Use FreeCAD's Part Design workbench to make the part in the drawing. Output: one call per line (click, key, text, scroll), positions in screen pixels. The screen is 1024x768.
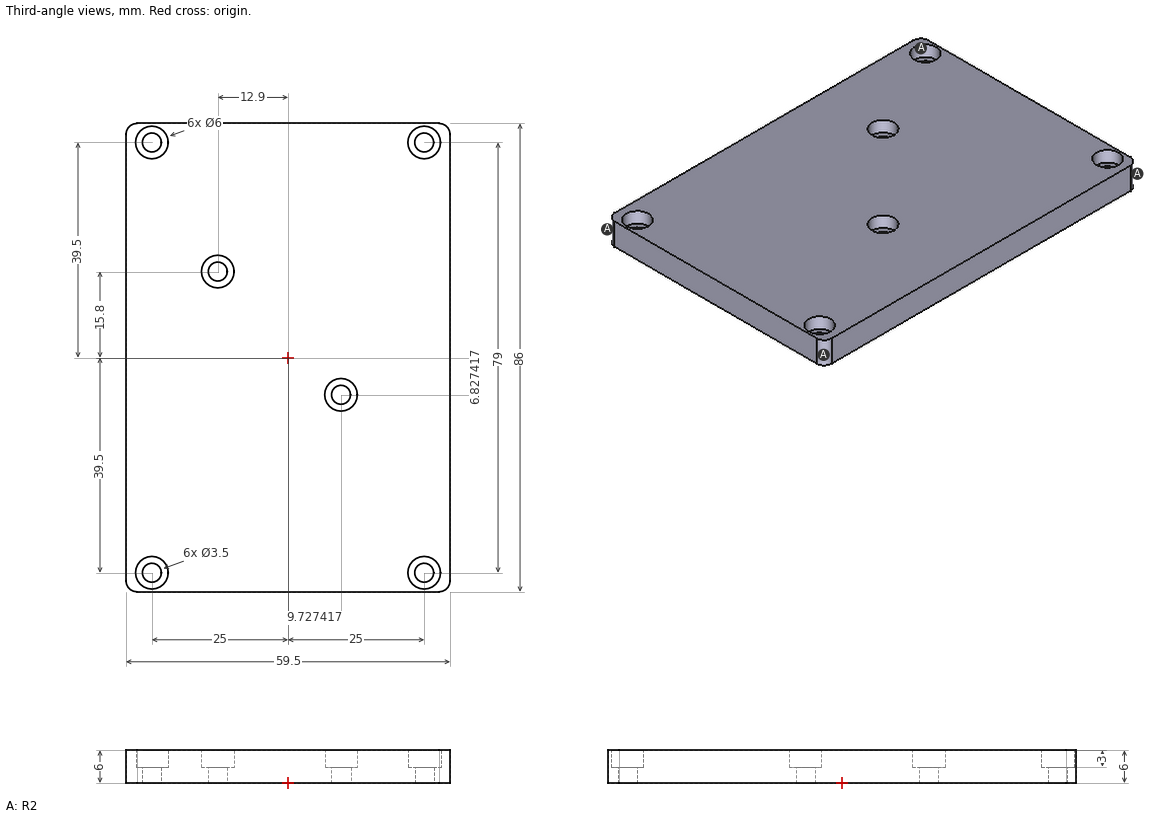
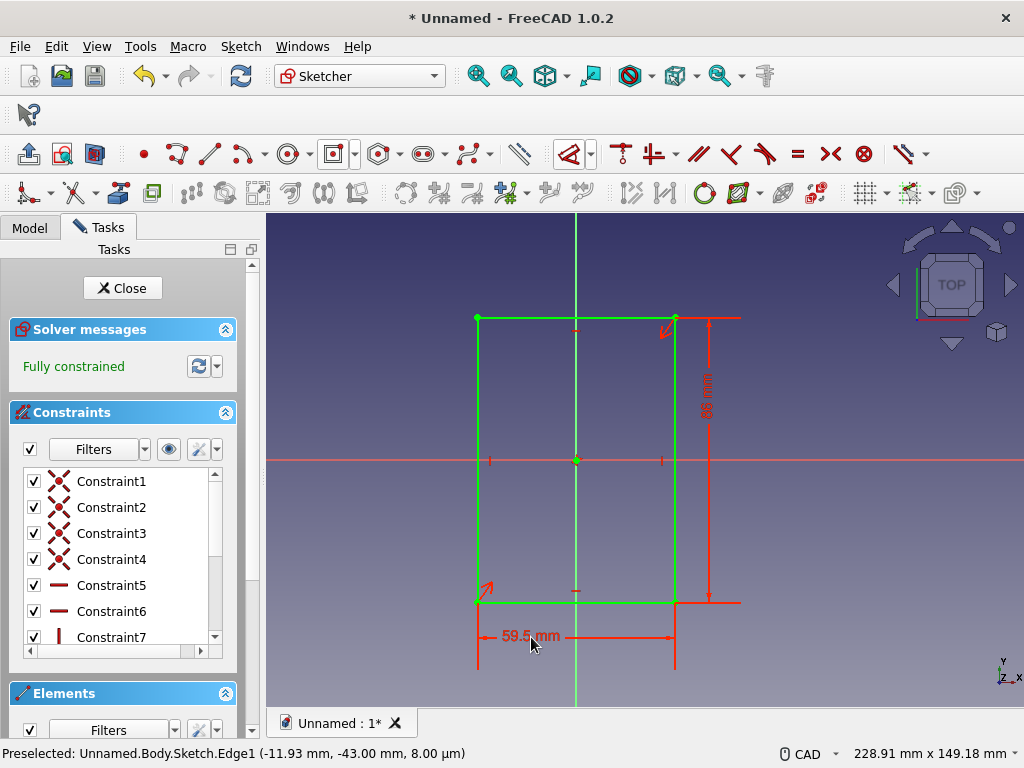
click(123, 288)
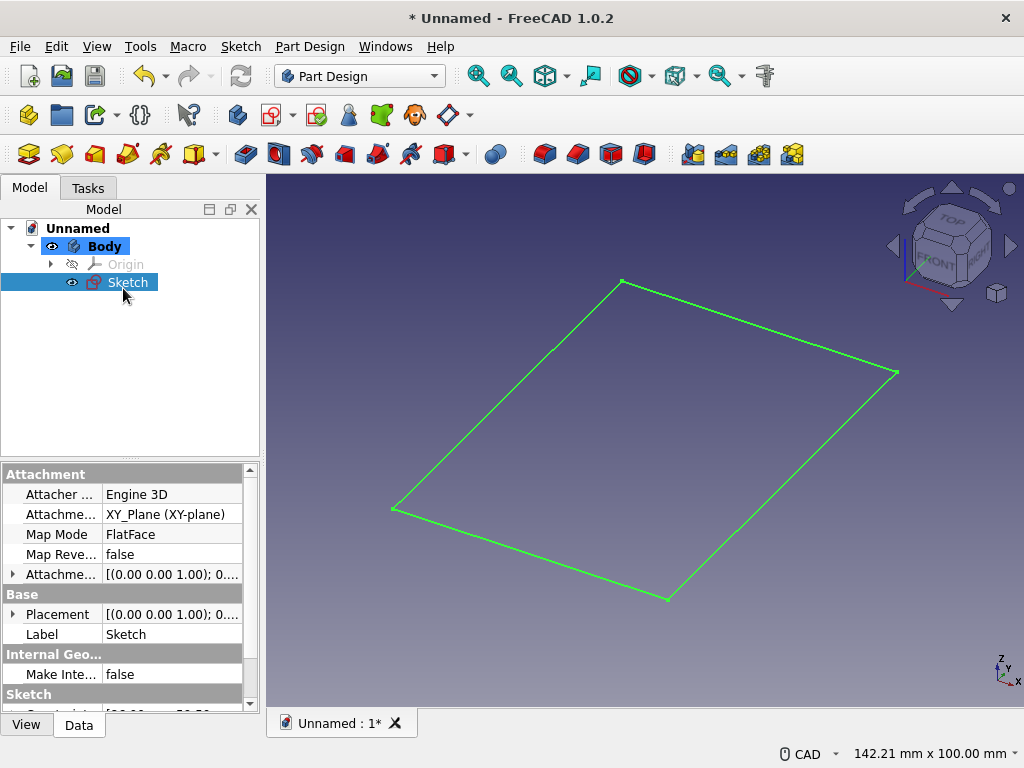
click(29, 154)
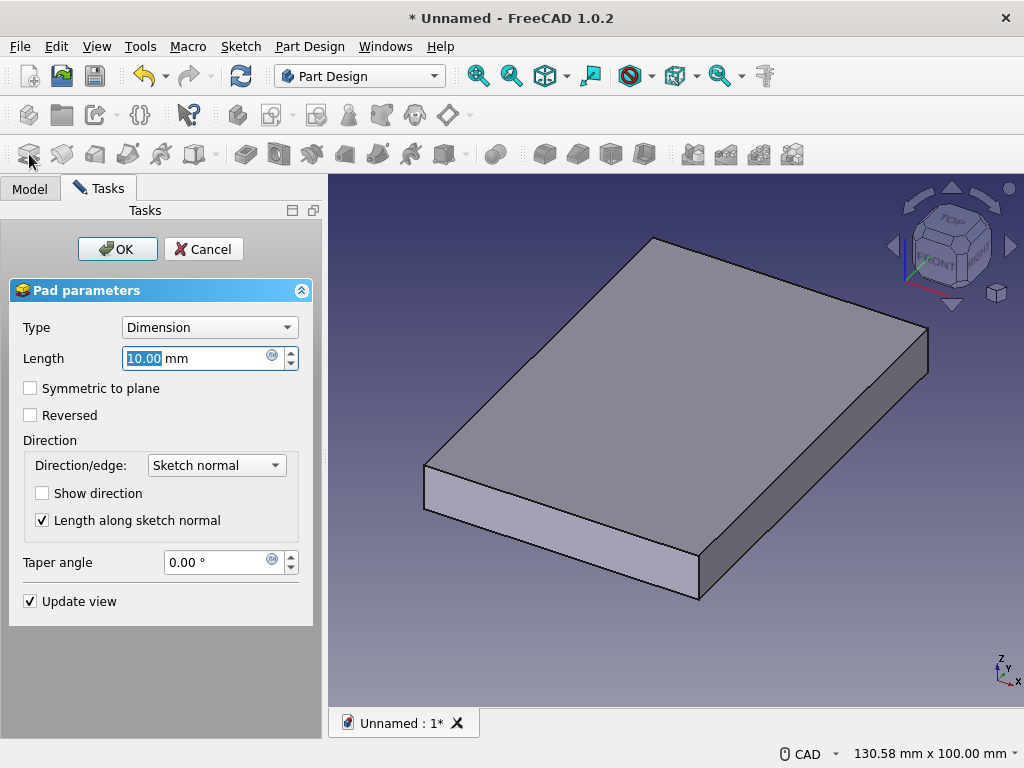
text(6)
key(Tab)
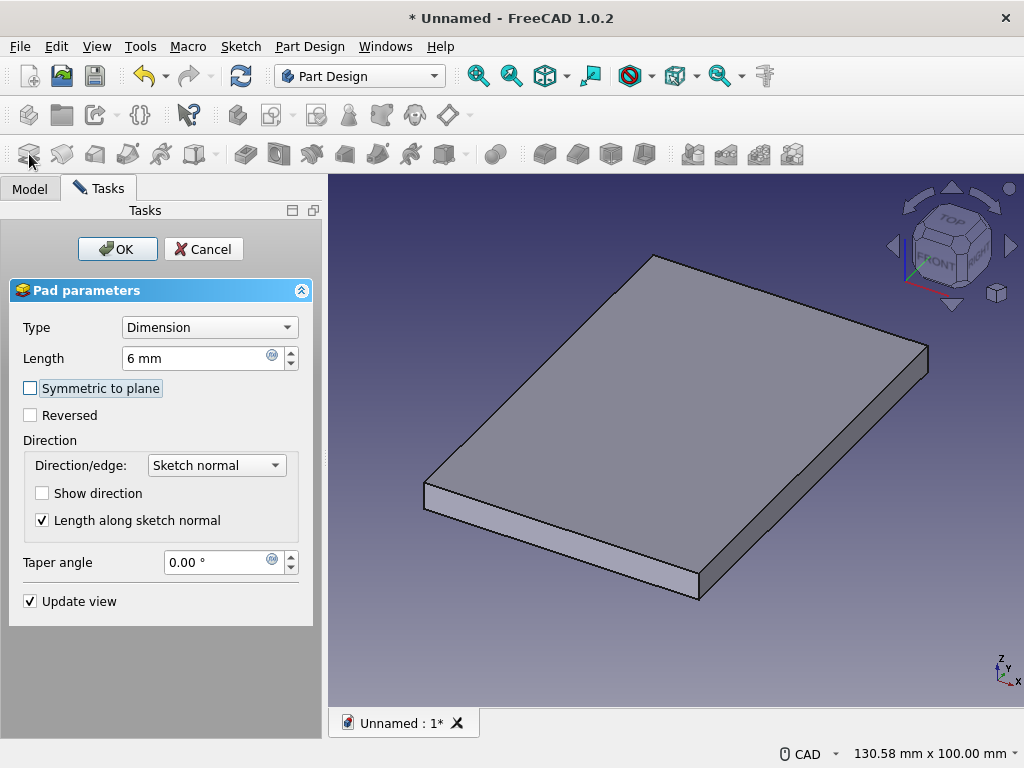
click(118, 249)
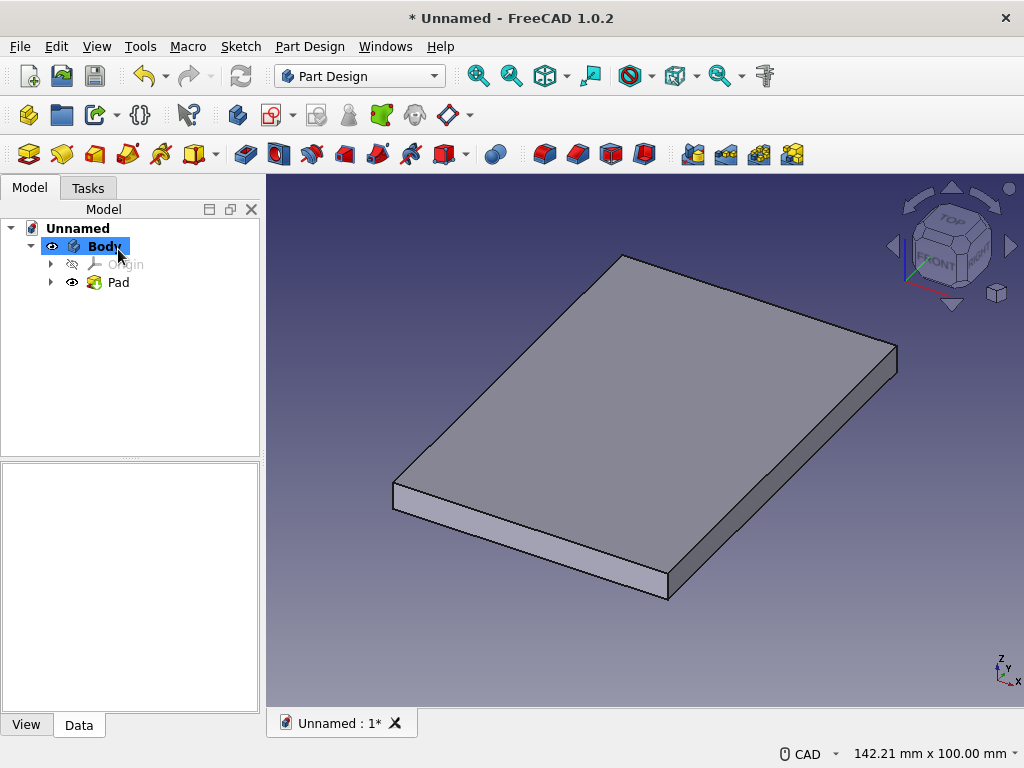
click(678, 381)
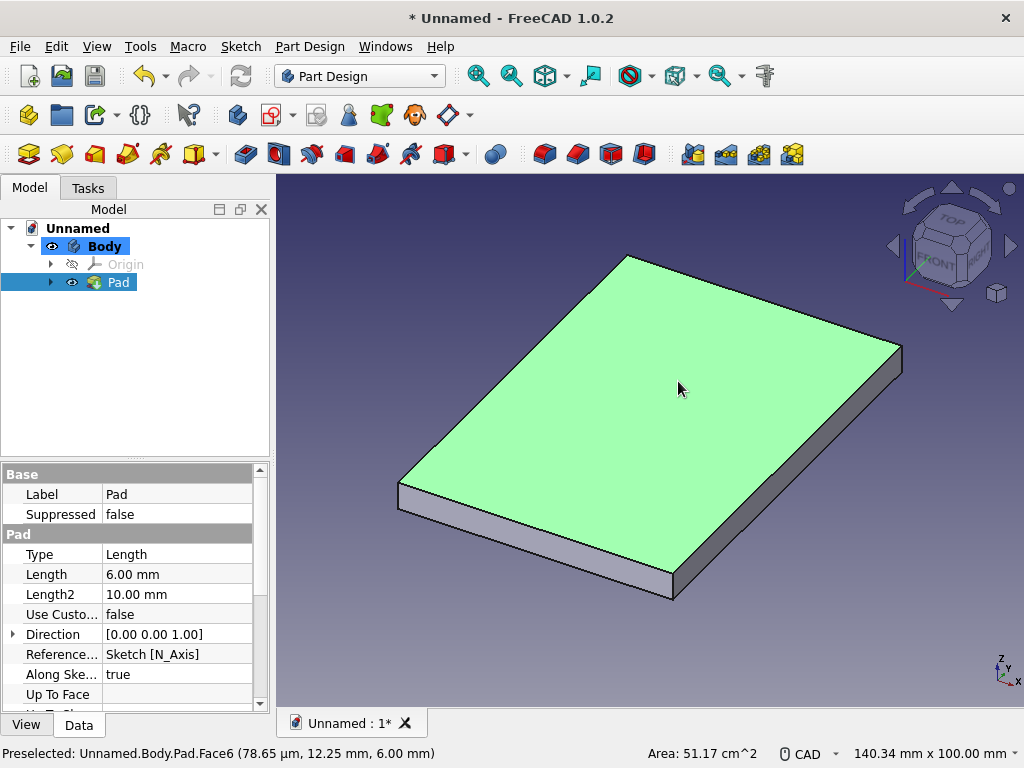
click(270, 116)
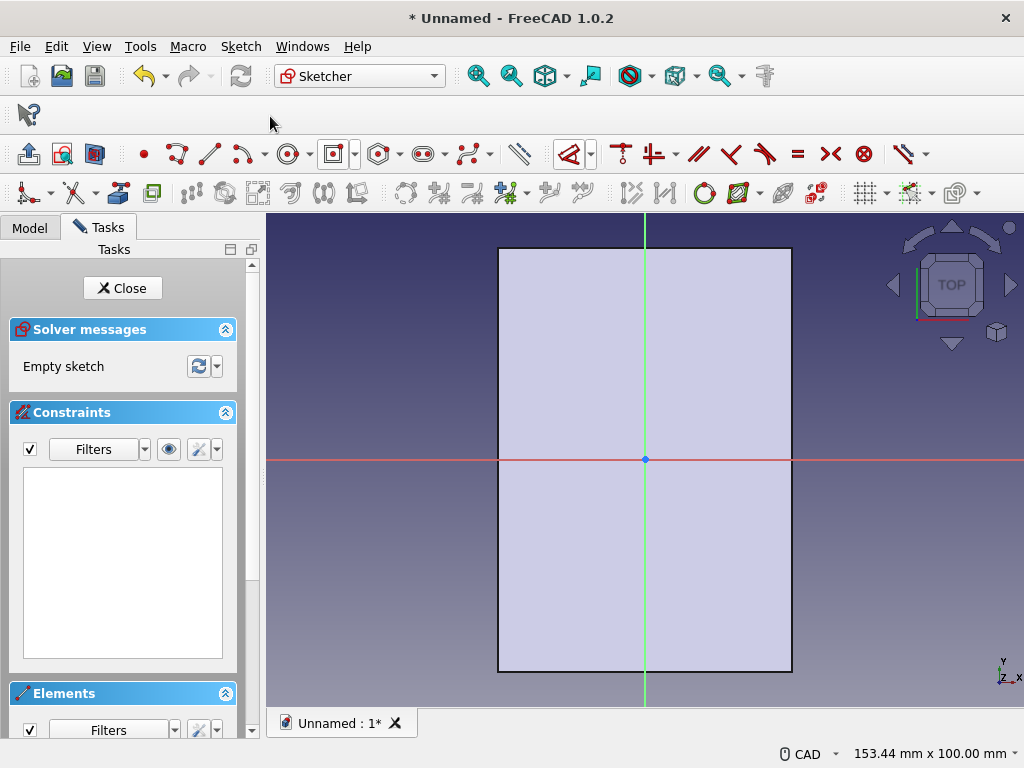
scroll(294, 460, down, 1)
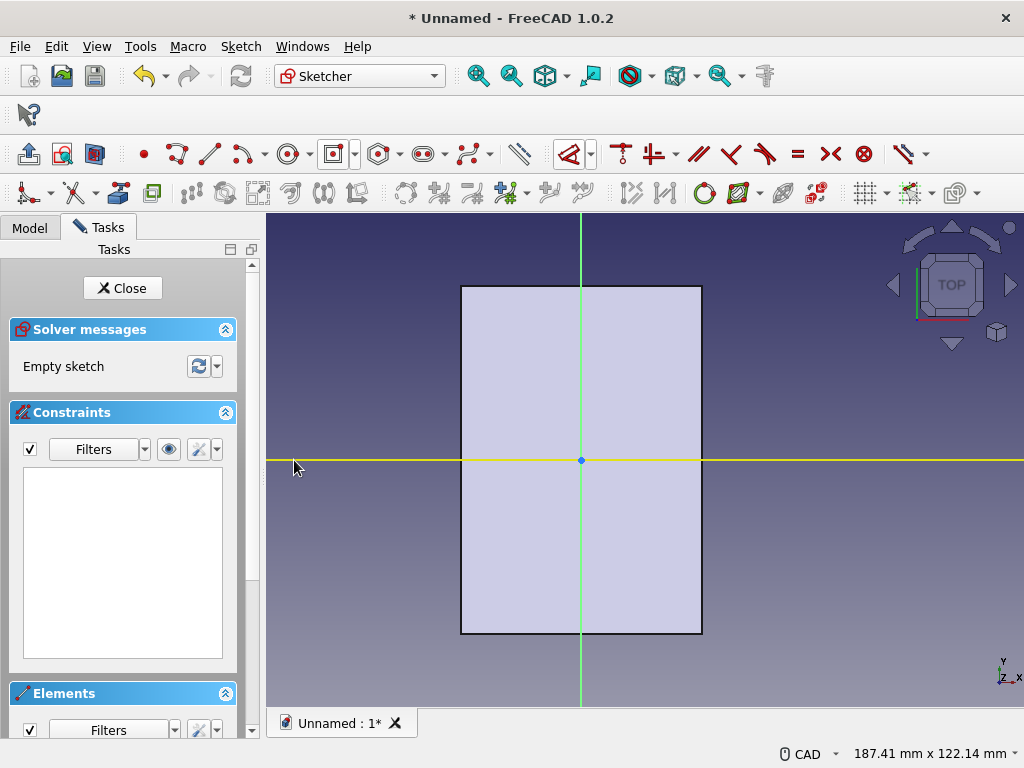
key(g)
key(c)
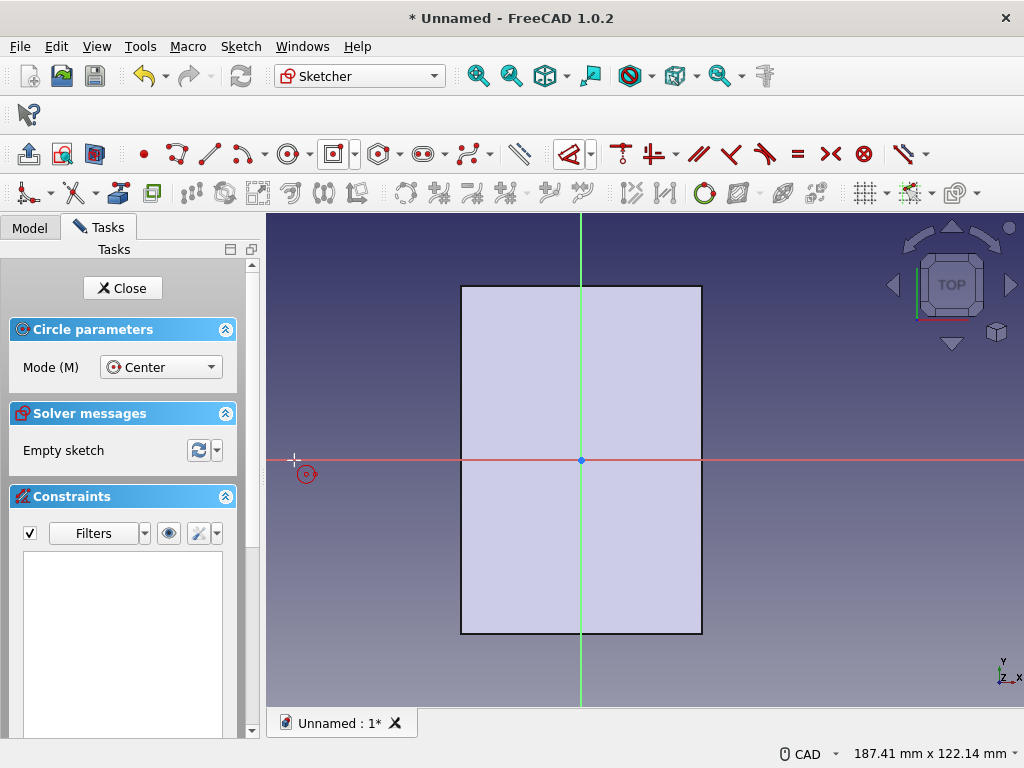
scroll(480, 620, up, 6)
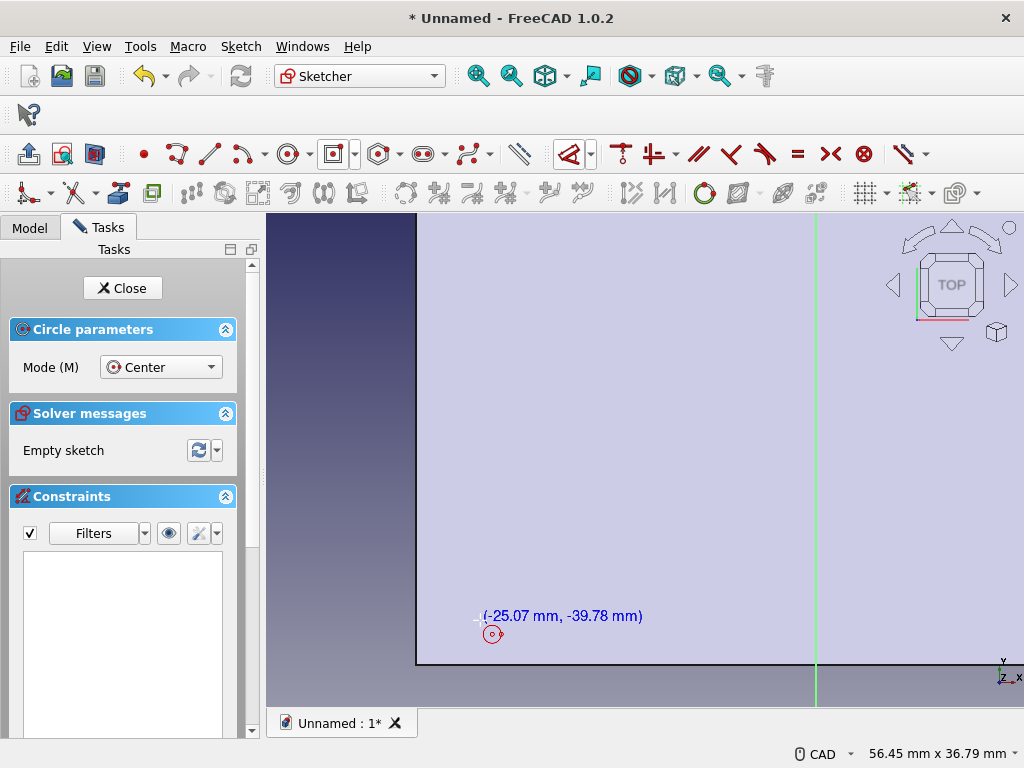
click(480, 618)
click(497, 601)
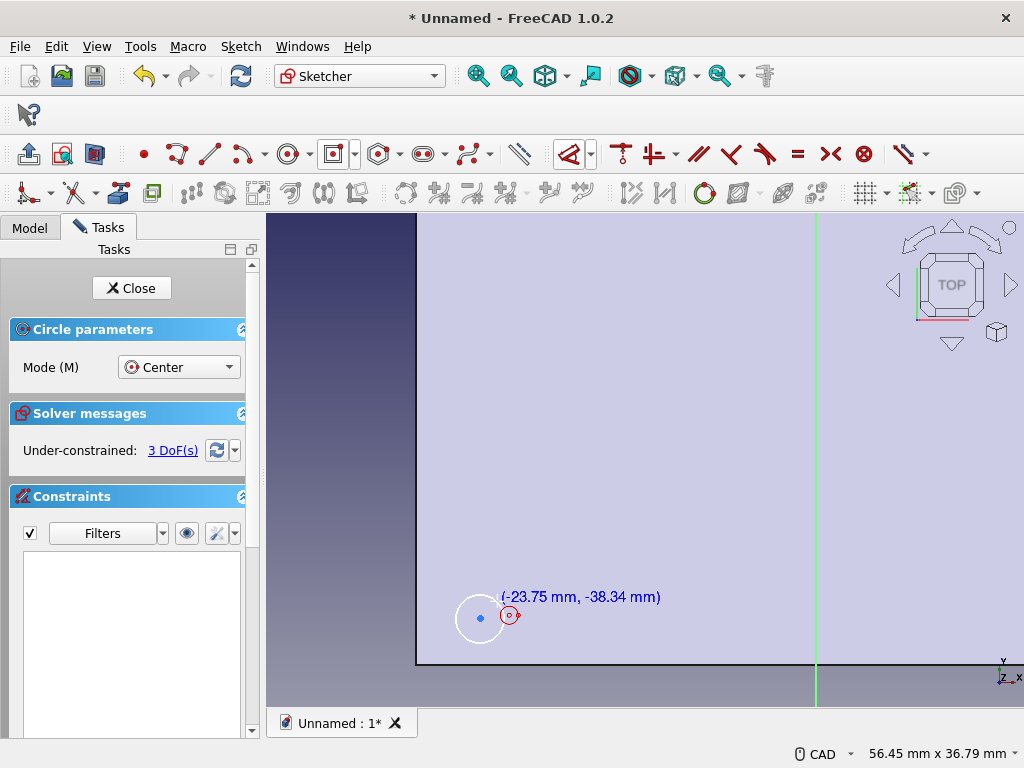
scroll(473, 621, down, 6)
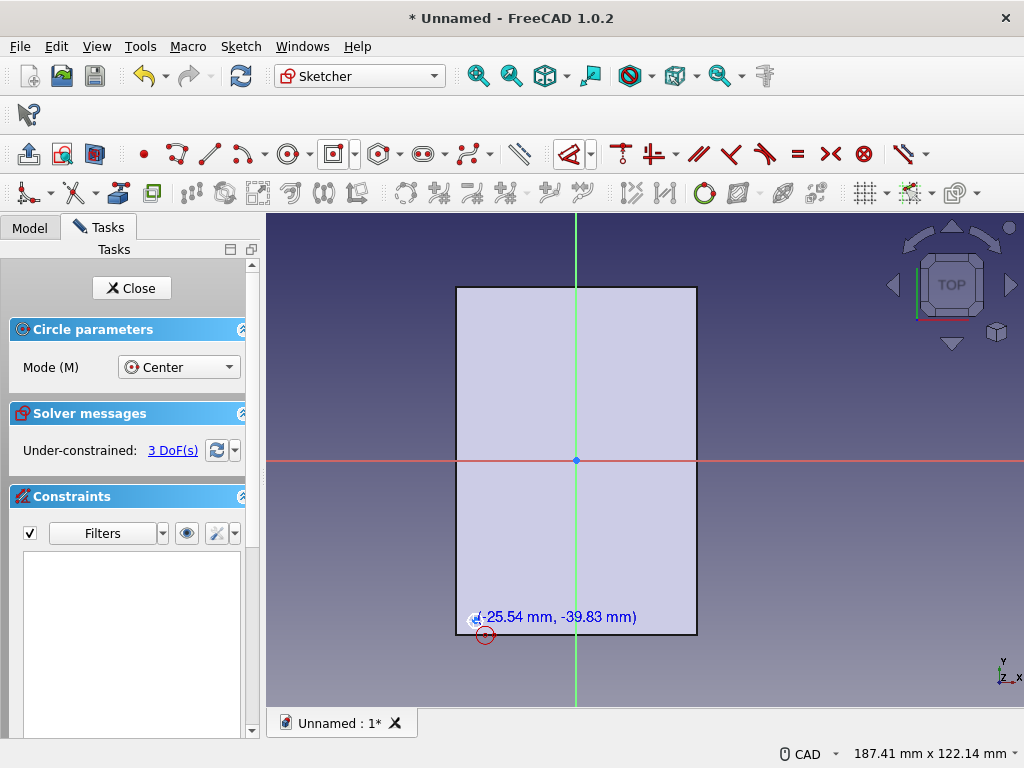
scroll(678, 621, up, 6)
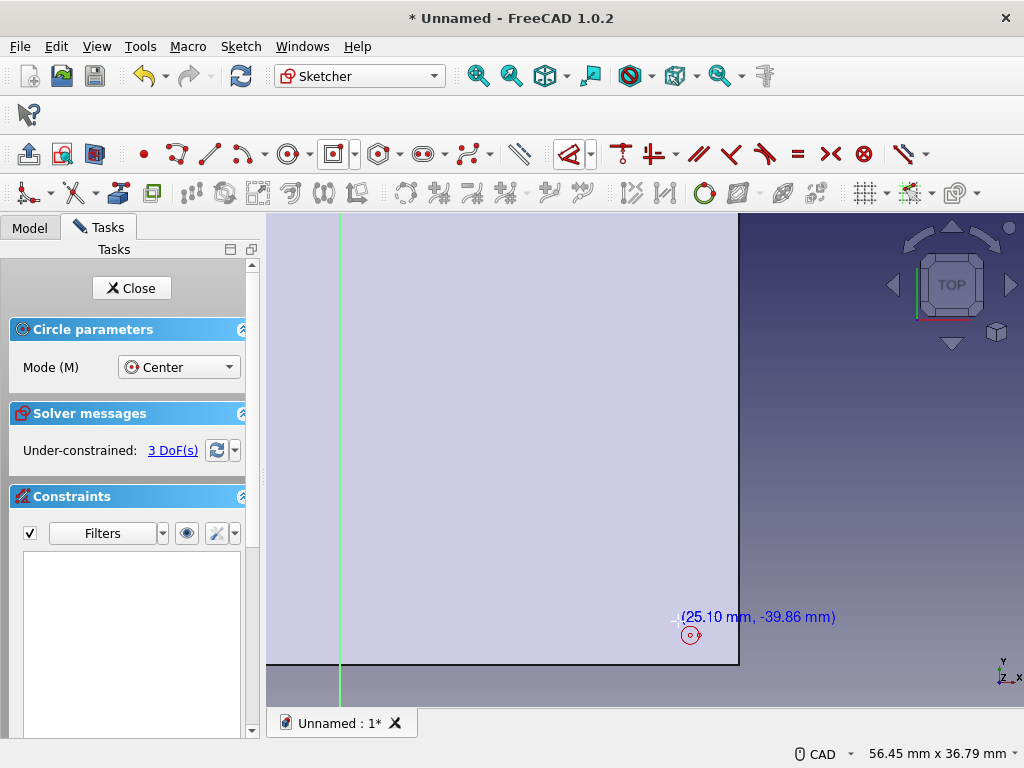
click(675, 618)
click(692, 601)